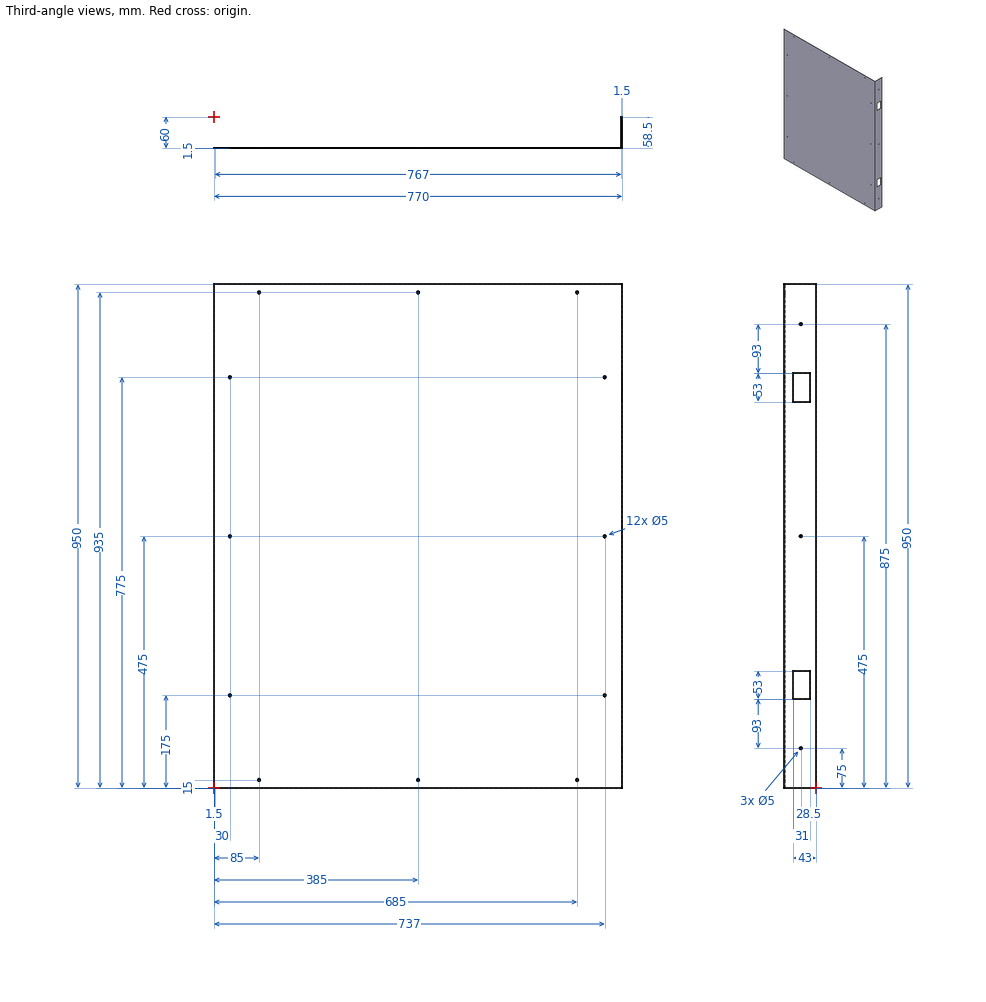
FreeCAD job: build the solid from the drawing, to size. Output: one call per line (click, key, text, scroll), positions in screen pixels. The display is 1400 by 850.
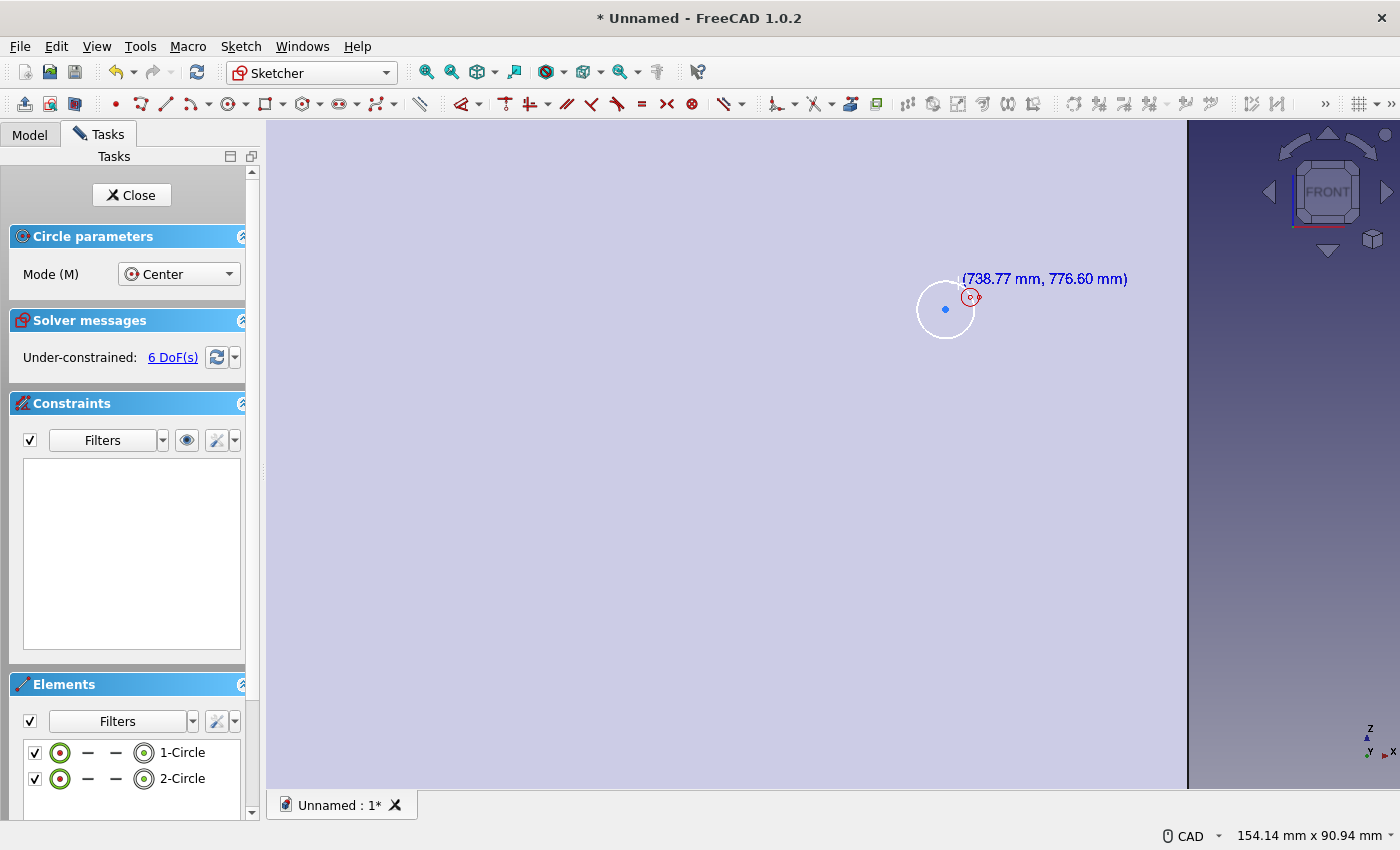
scroll(928, 319, down, 14)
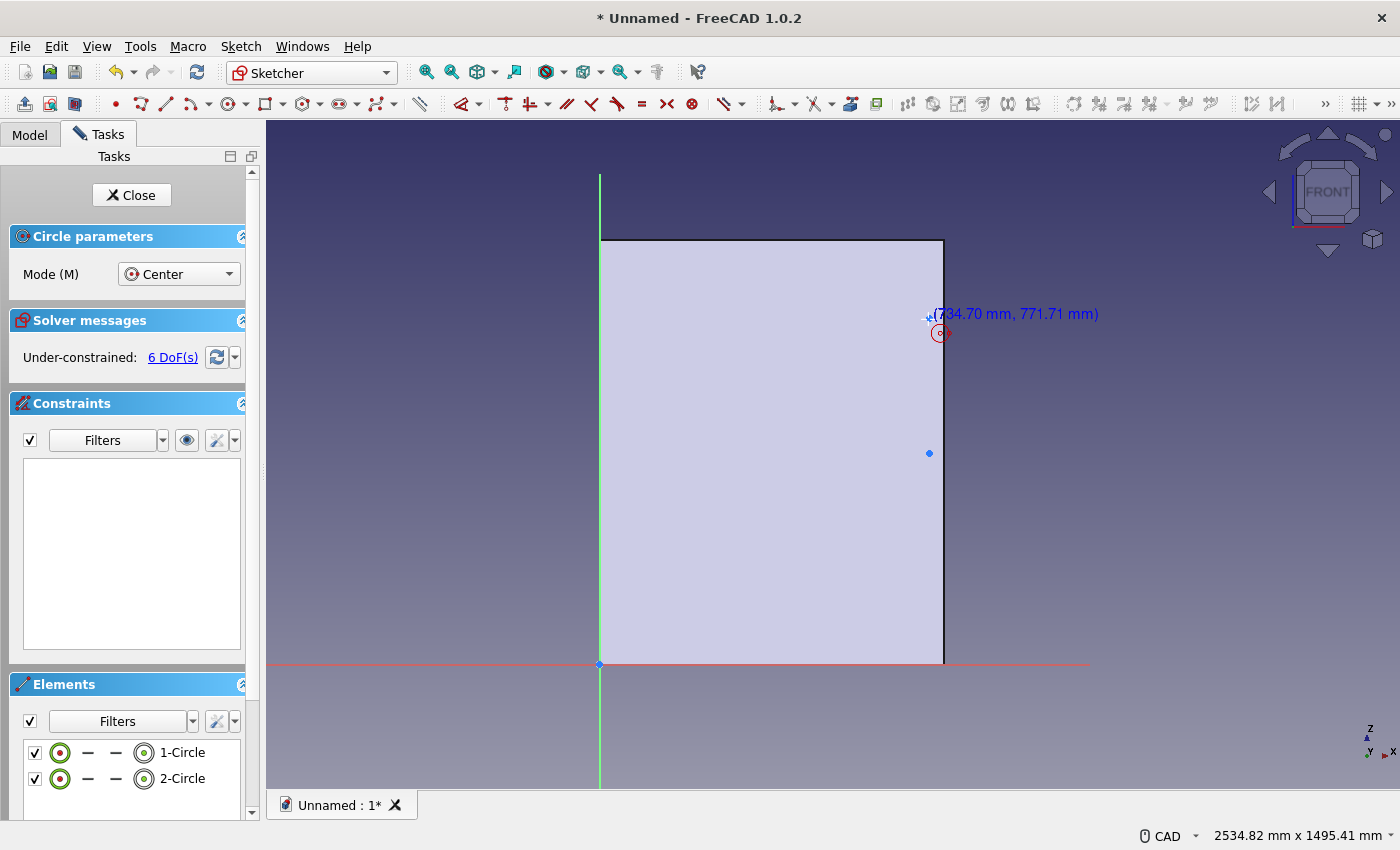
scroll(930, 586, up, 16)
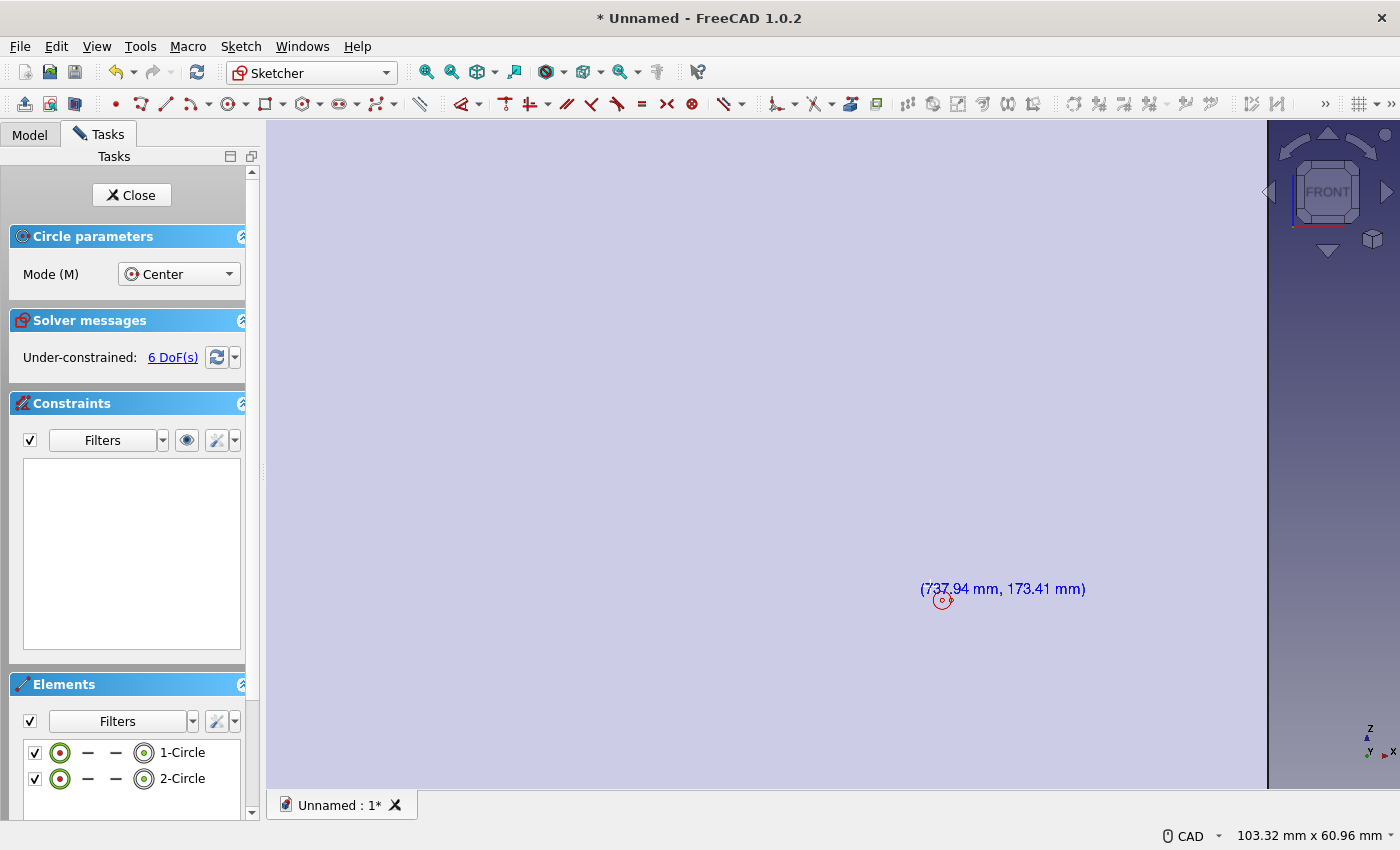
scroll(968, 617, down, 15)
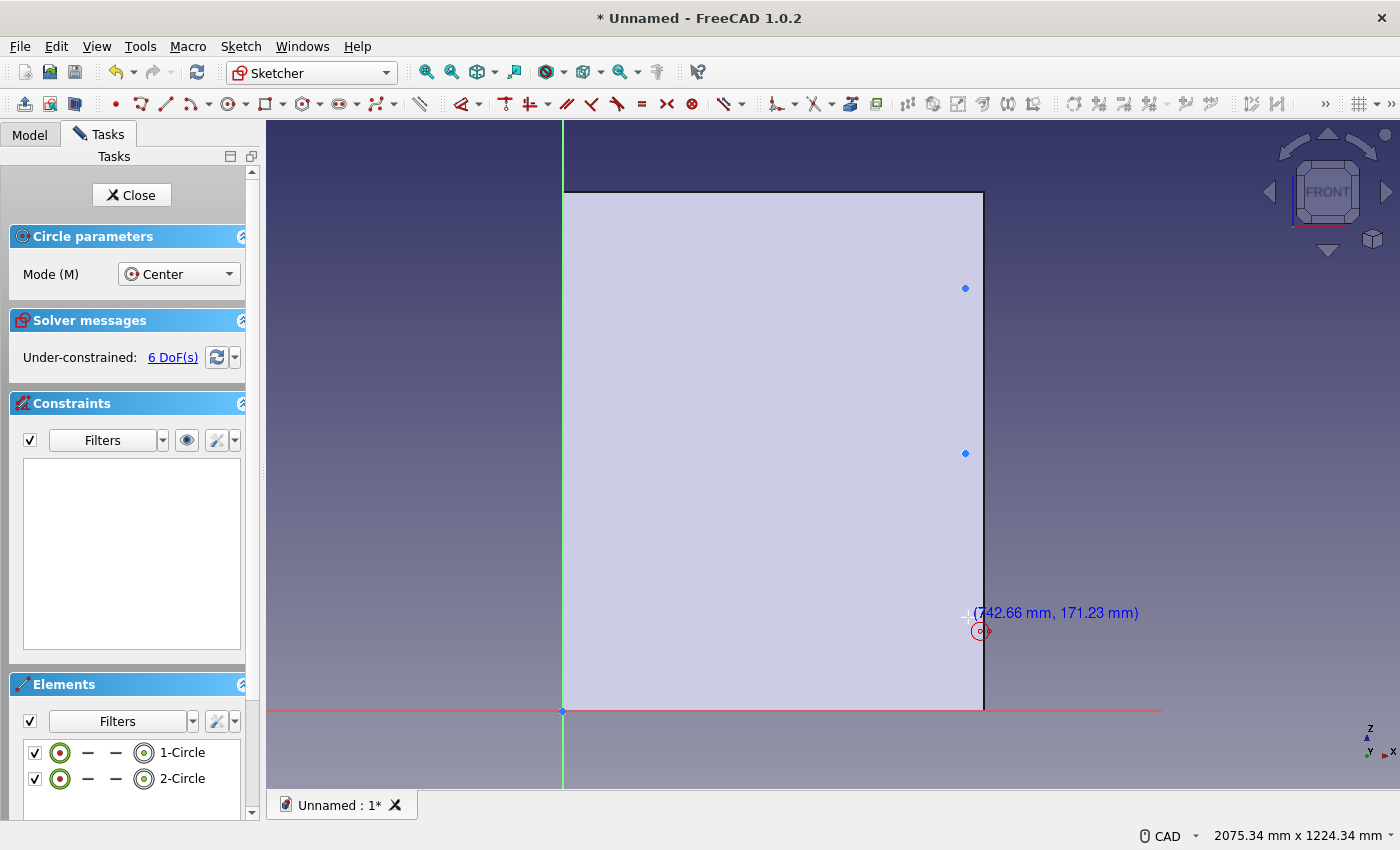
click(965, 616)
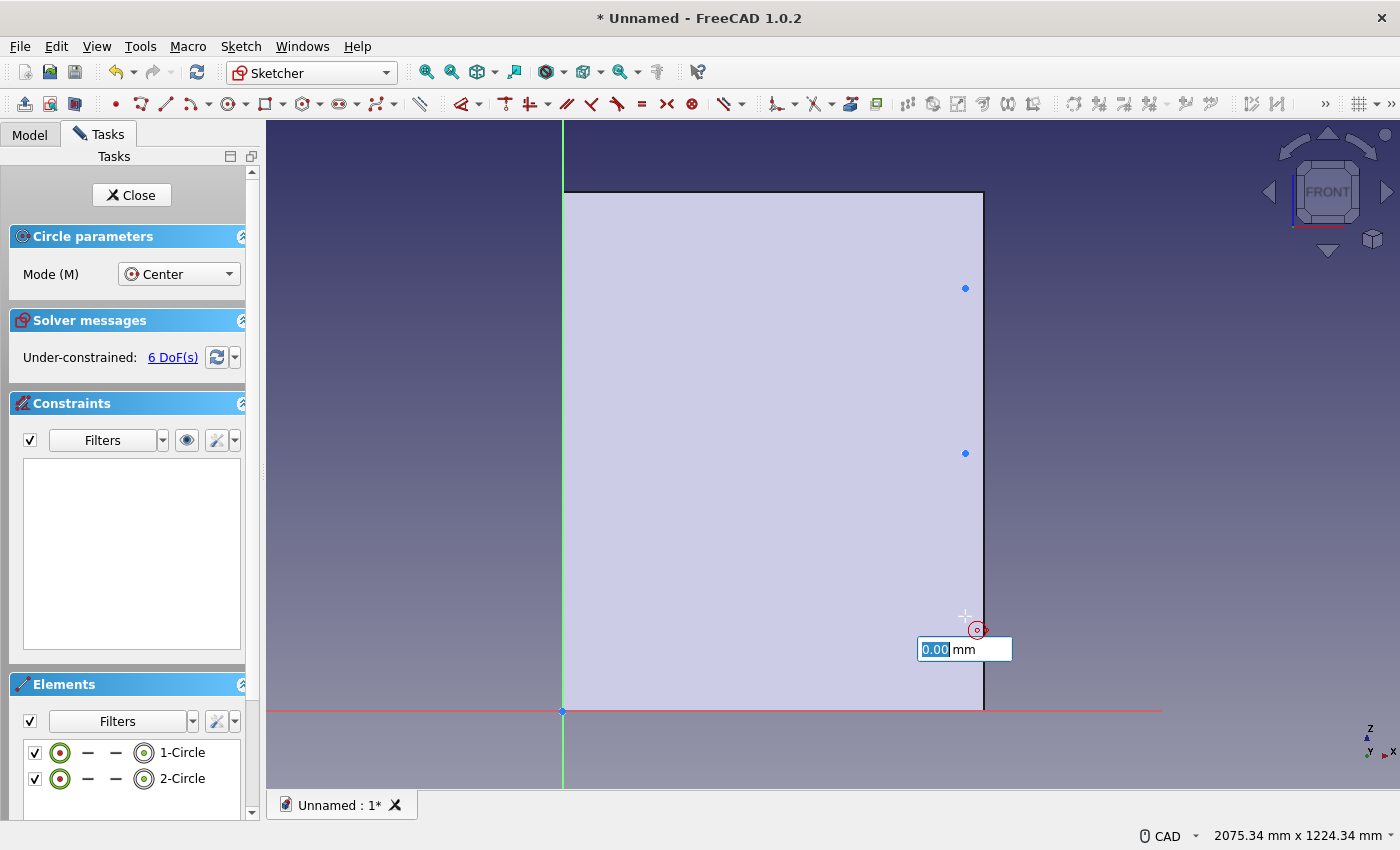
scroll(966, 615, up, 13)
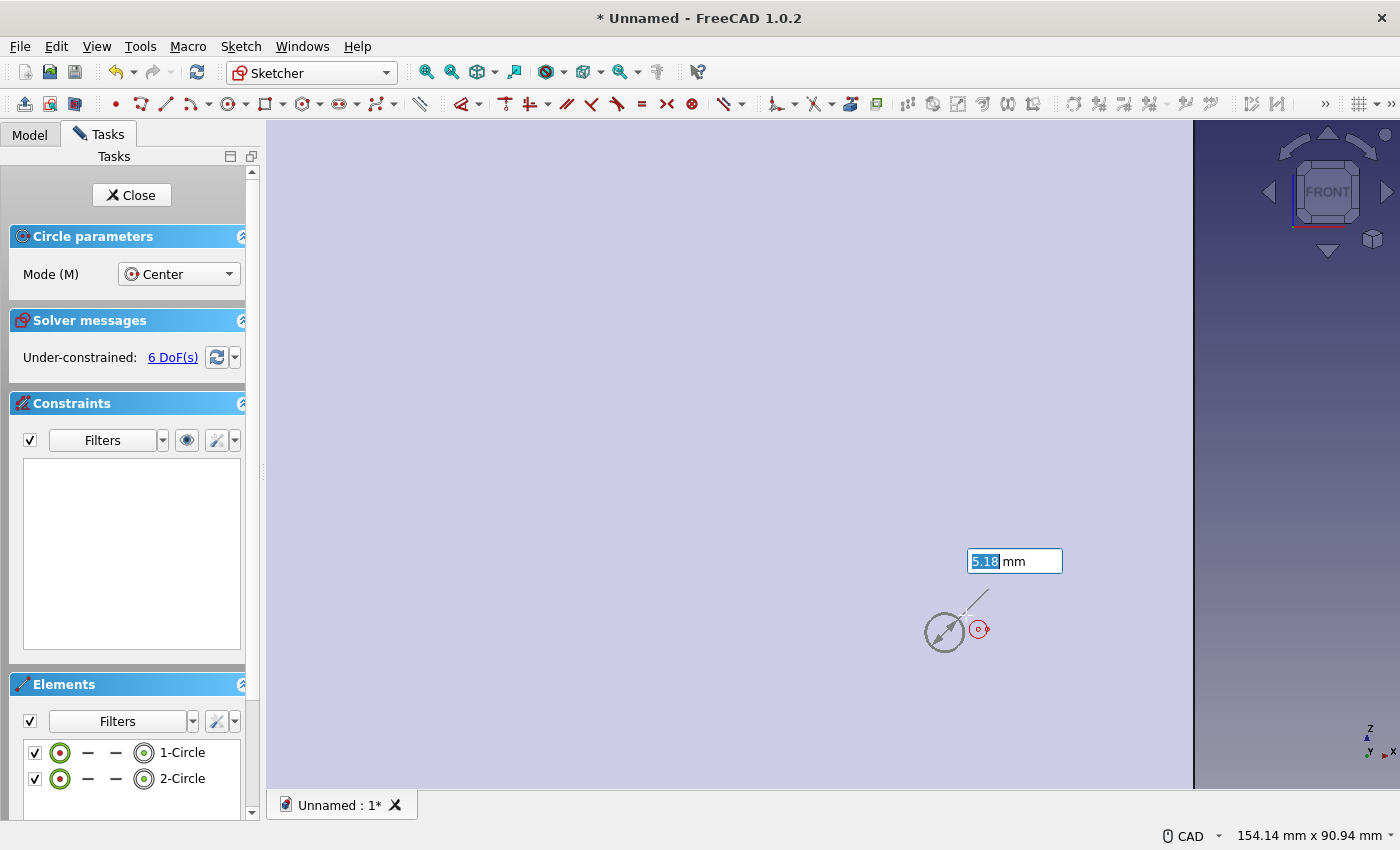
click(965, 602)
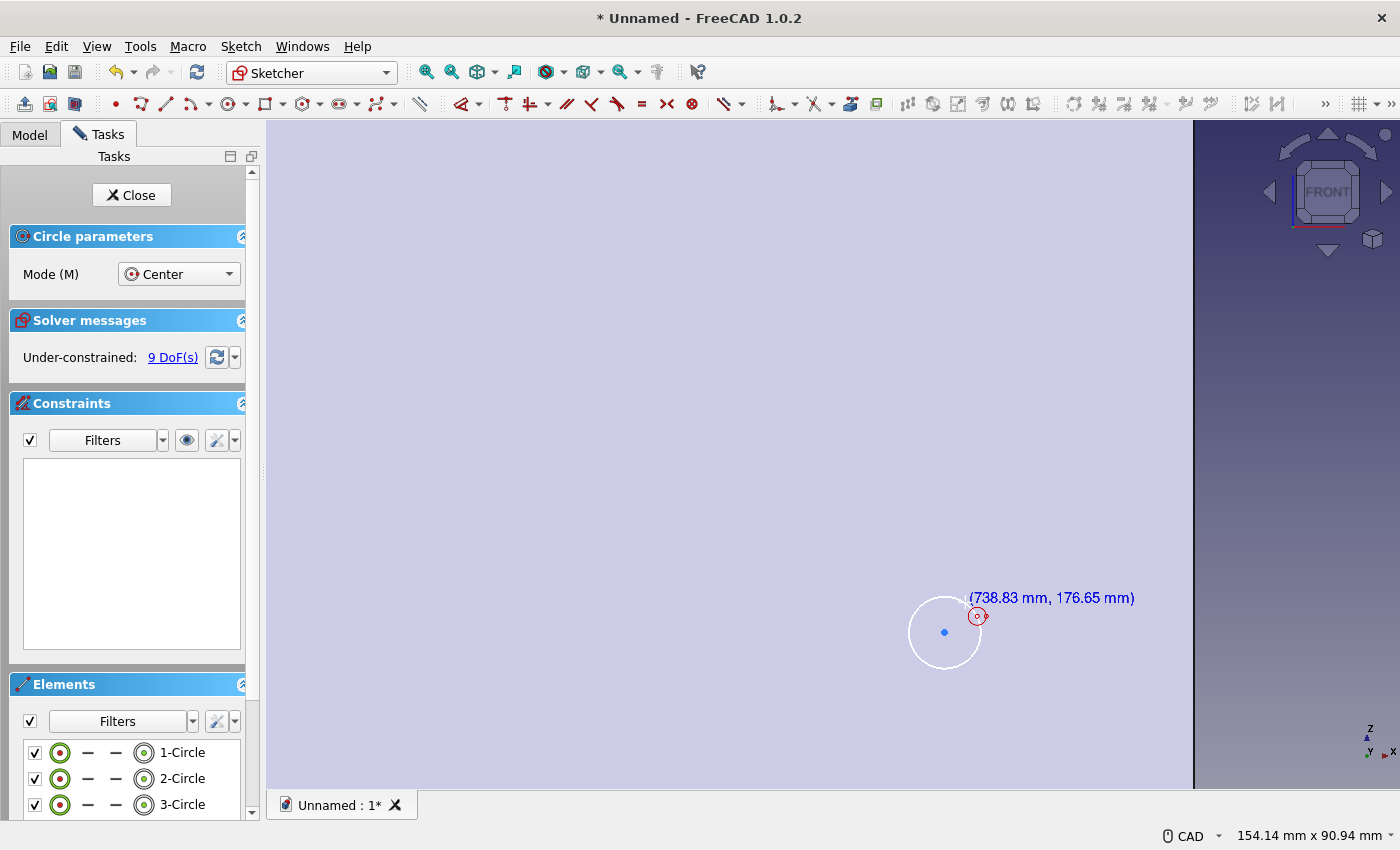
scroll(927, 584, down, 14)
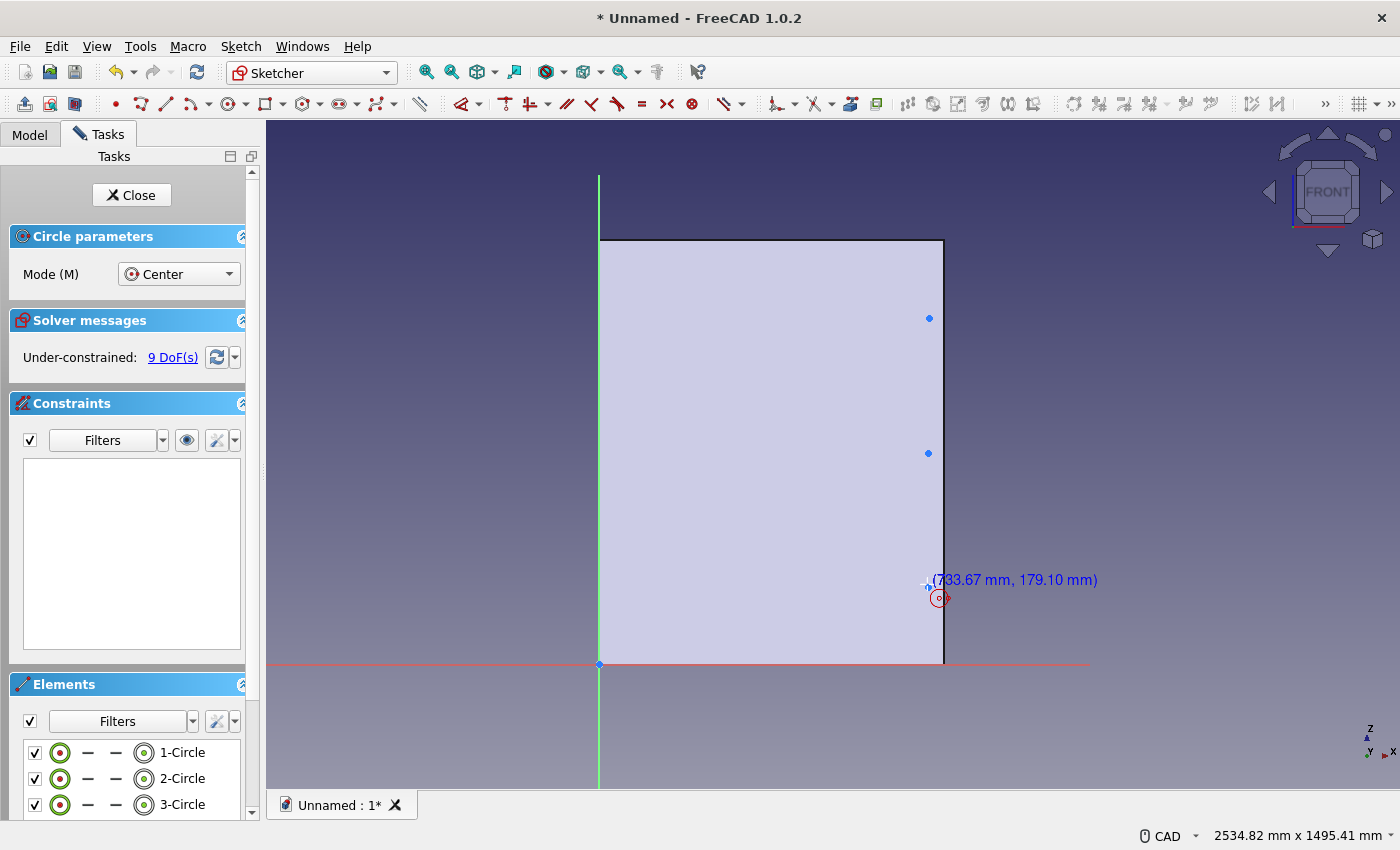
scroll(613, 318, up, 16)